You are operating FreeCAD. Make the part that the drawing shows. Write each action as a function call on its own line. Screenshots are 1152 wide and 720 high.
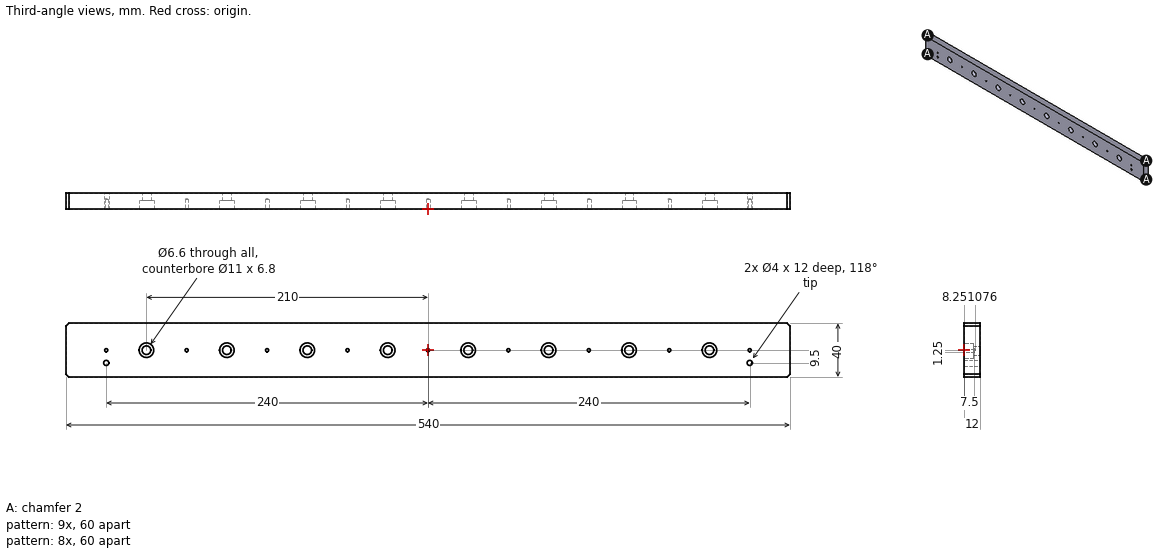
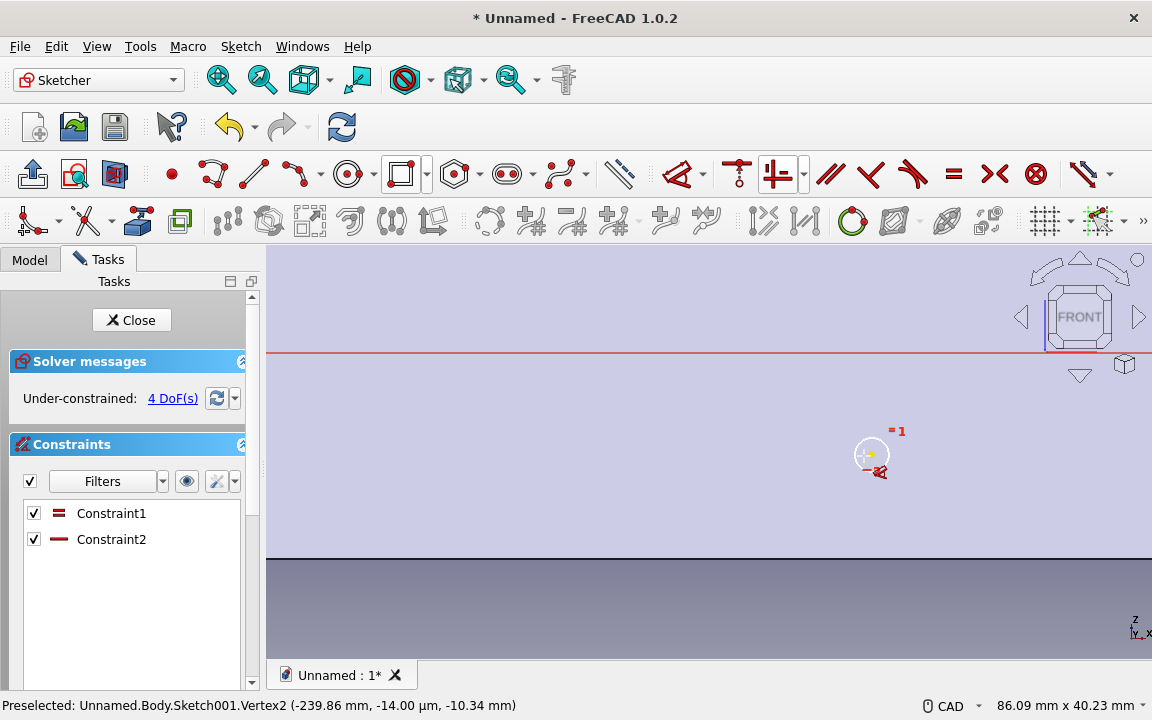
click(855, 454)
click(823, 452)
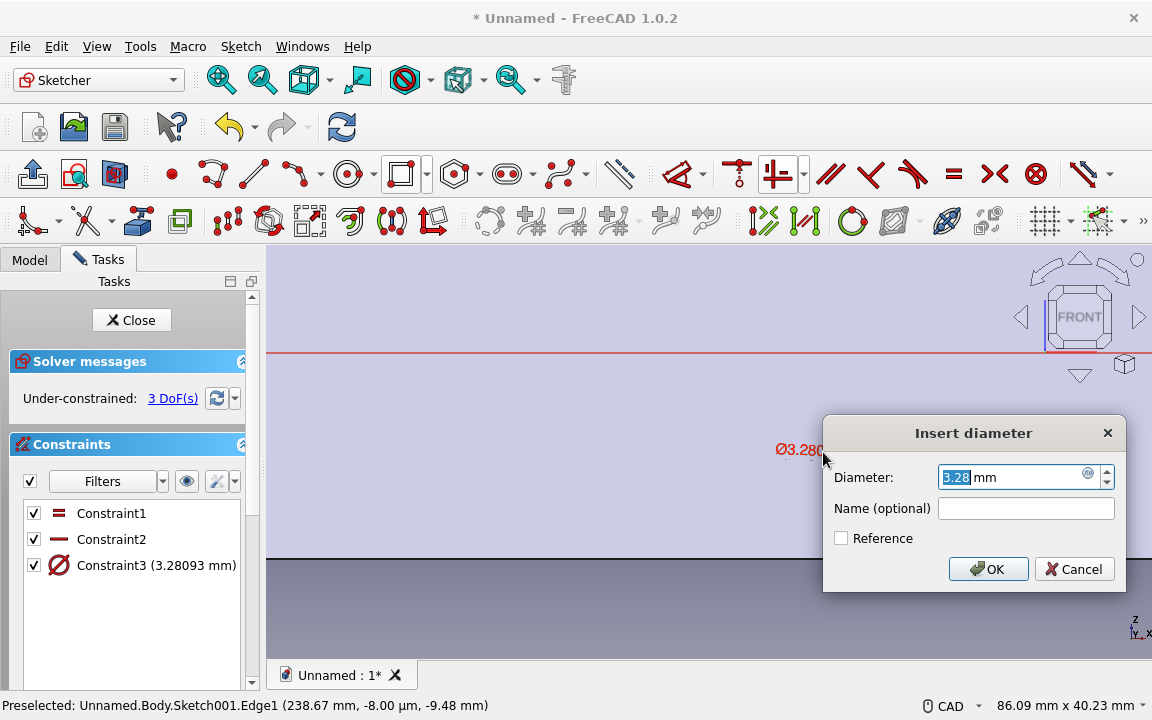
text(4)
key(Return)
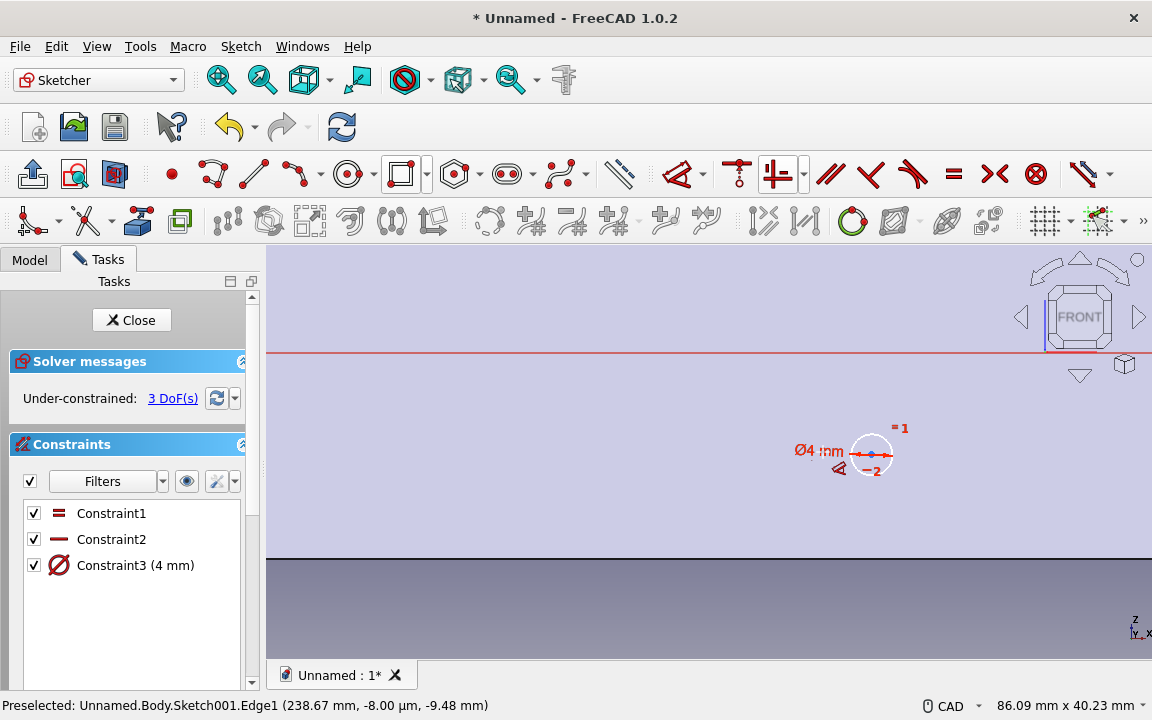
scroll(864, 456, down, 12)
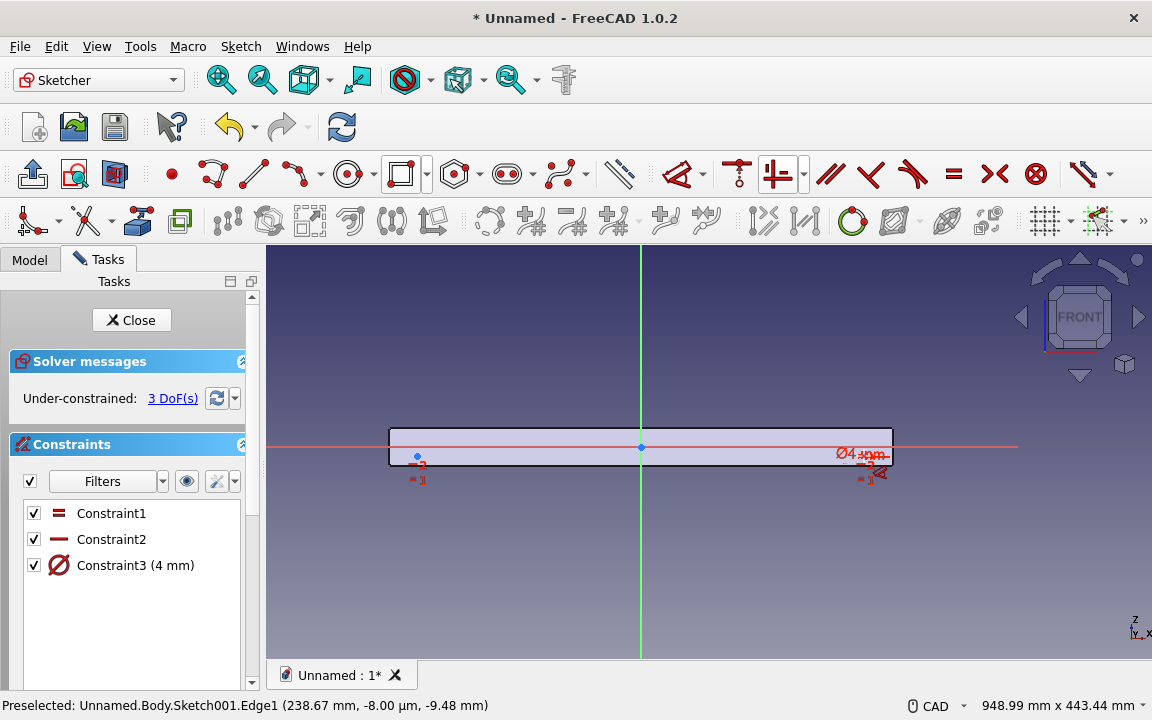
click(865, 456)
click(753, 413)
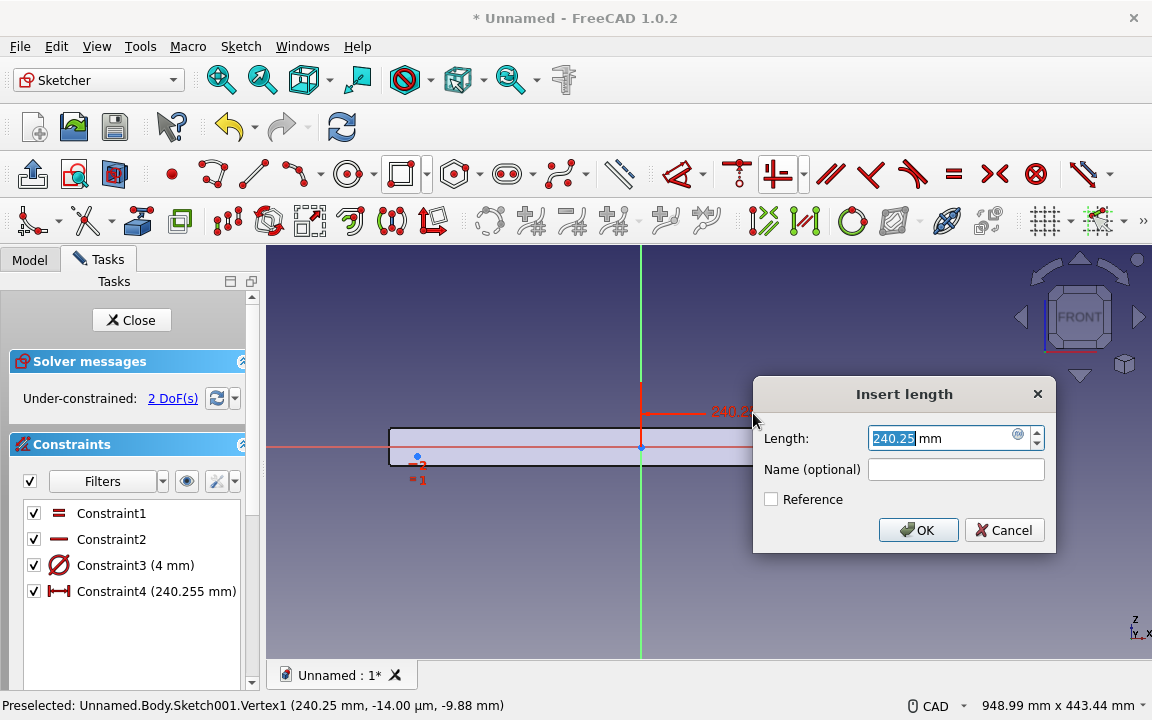
text(240)
key(Return)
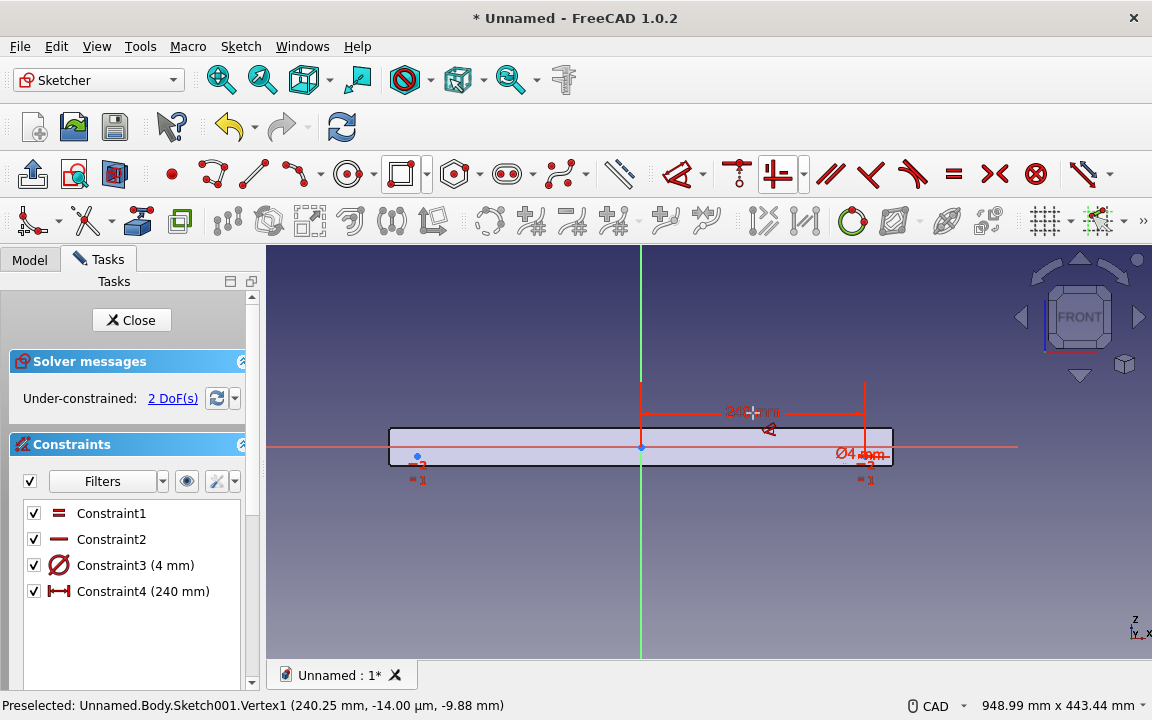
scroll(865, 456, up, 8)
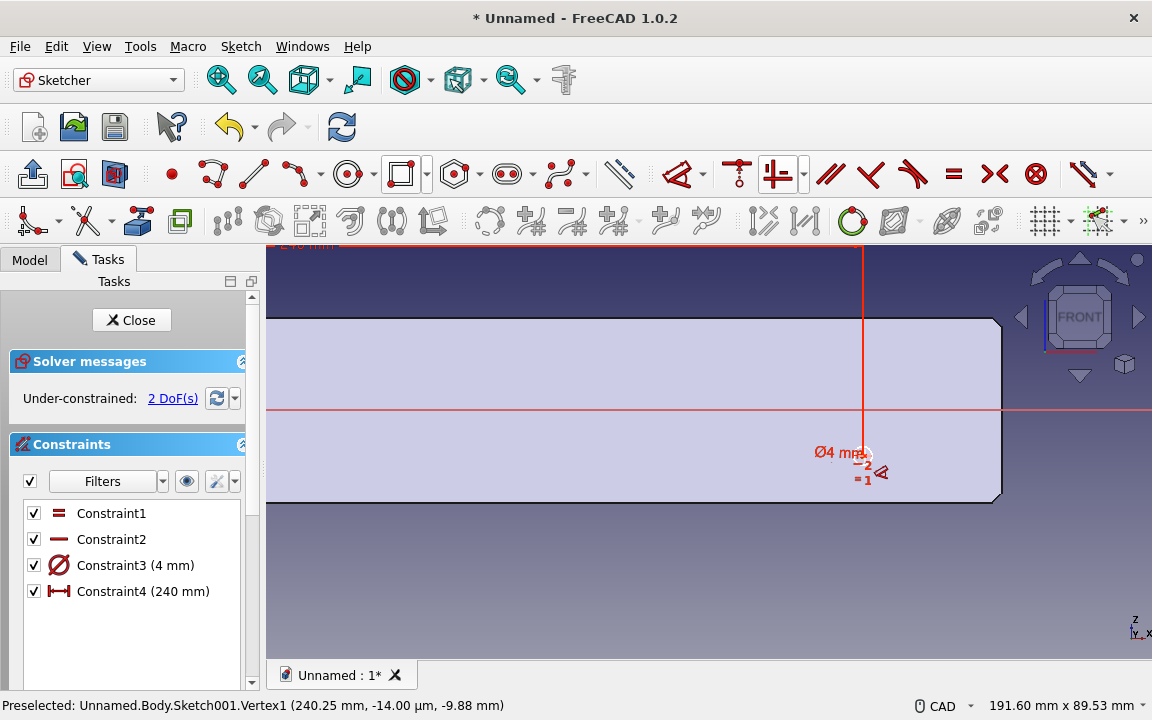
click(863, 456)
click(897, 433)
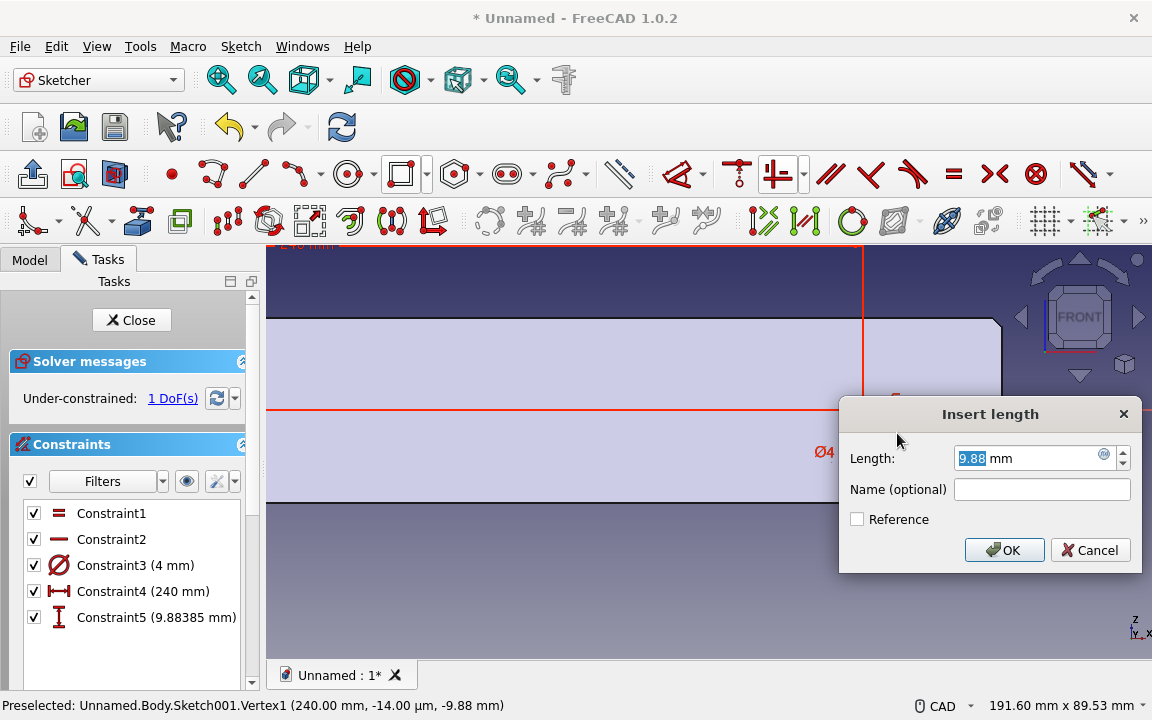
text(9.5)
key(Return)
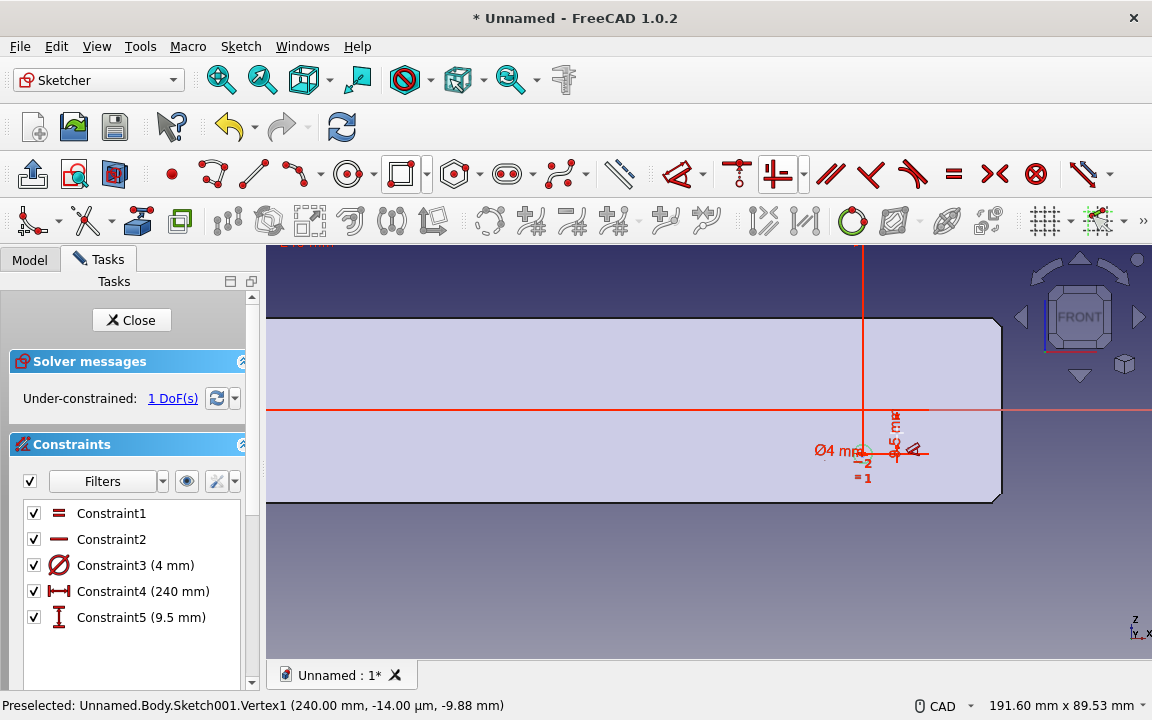
scroll(865, 456, down, 8)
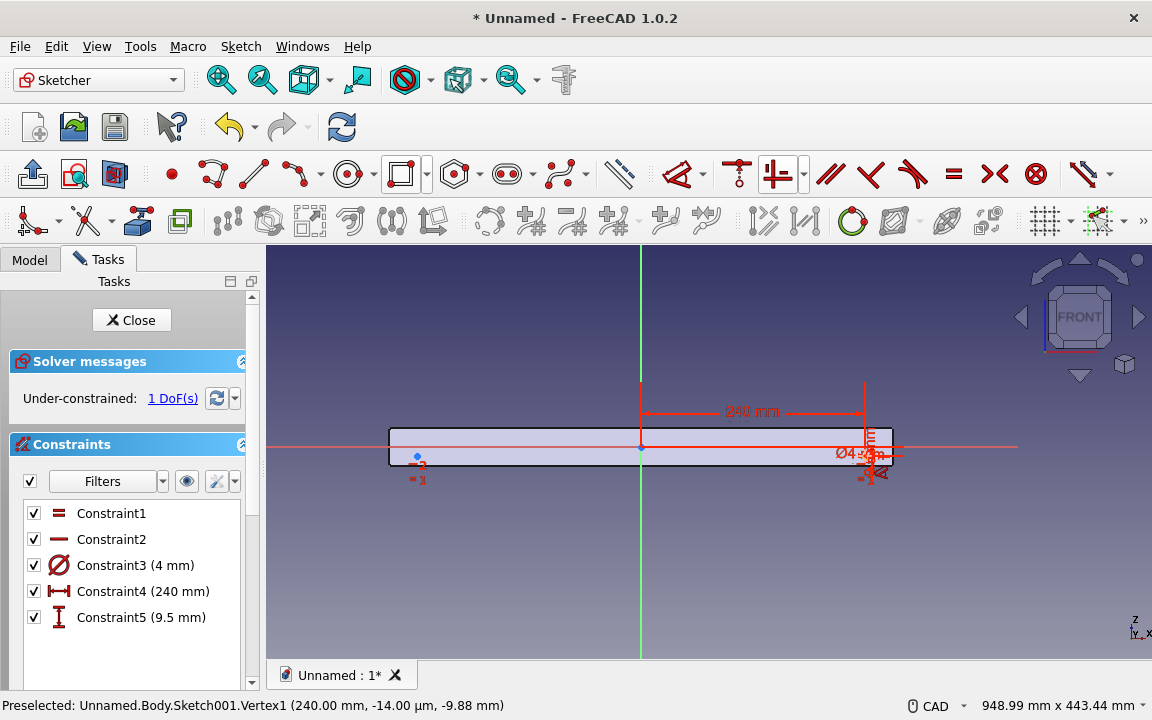
click(417, 456)
click(529, 413)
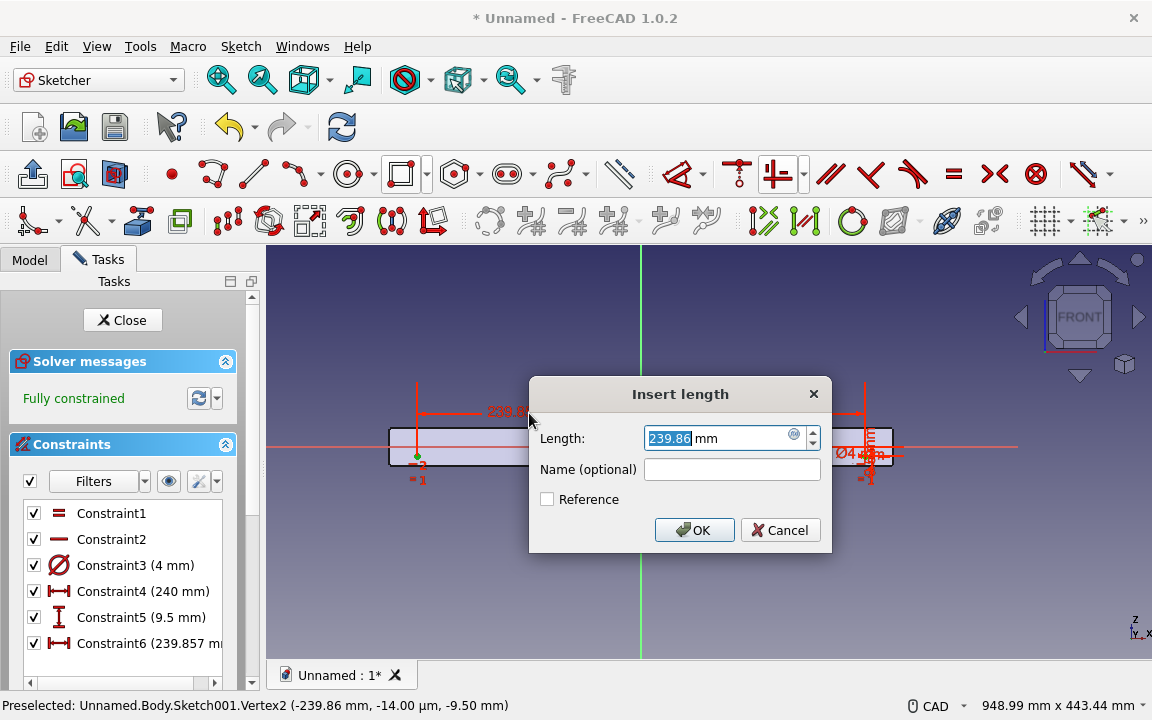
text(240)
key(Return)
key(Escape)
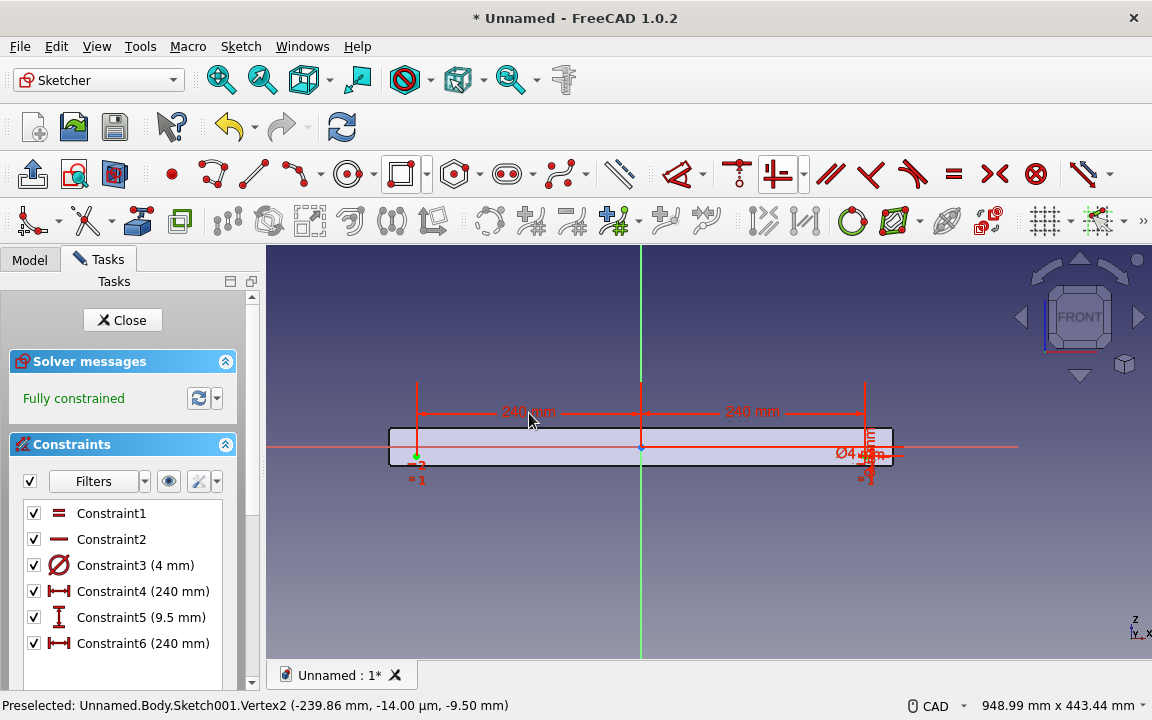
click(123, 320)